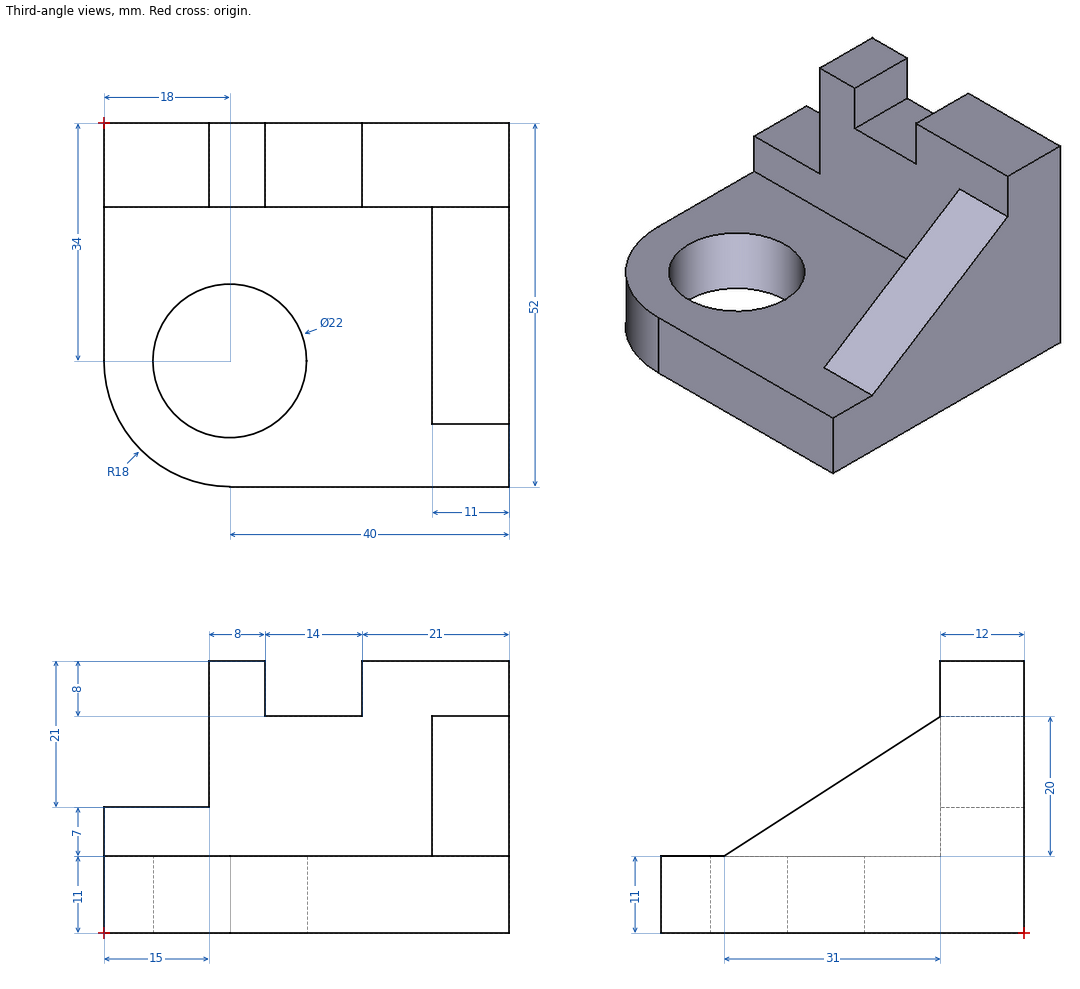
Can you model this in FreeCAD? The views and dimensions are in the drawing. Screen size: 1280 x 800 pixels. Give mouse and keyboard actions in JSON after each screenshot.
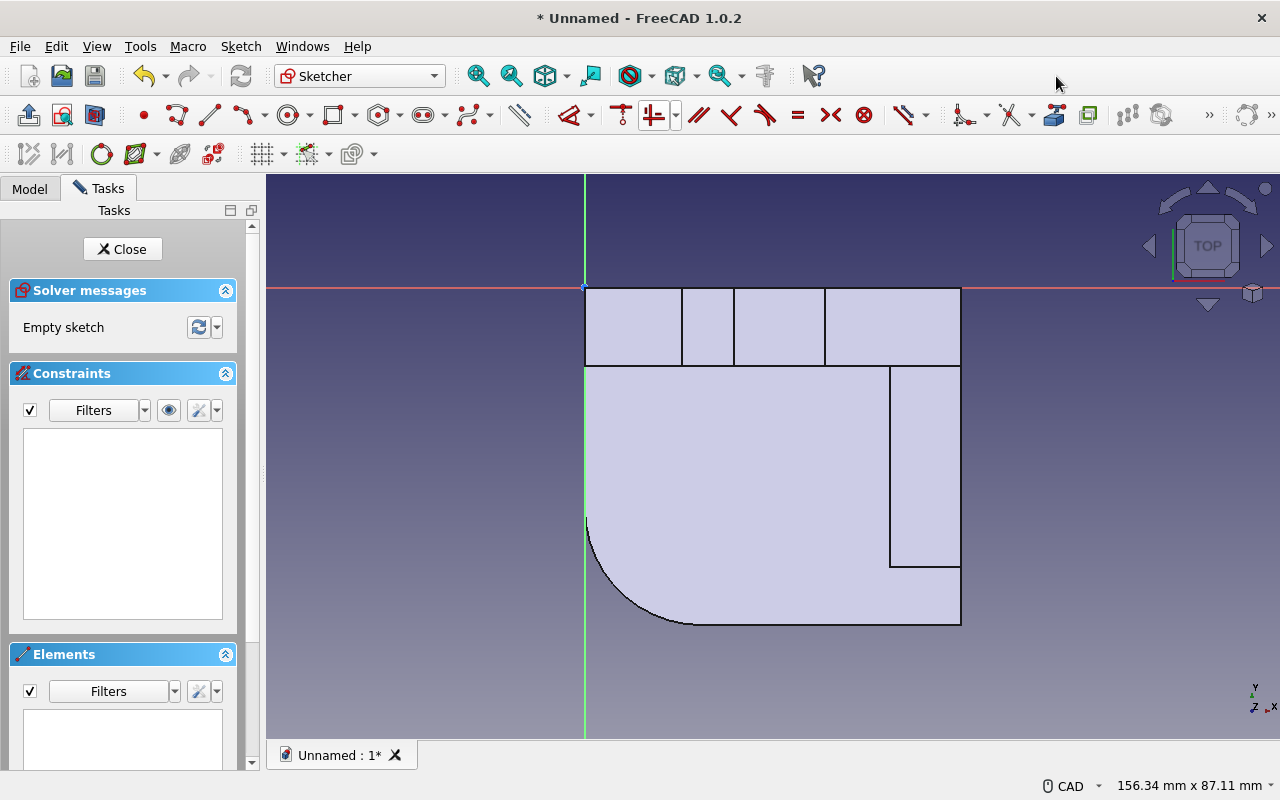
{"action": "left_click", "coordinate": [95, 116]}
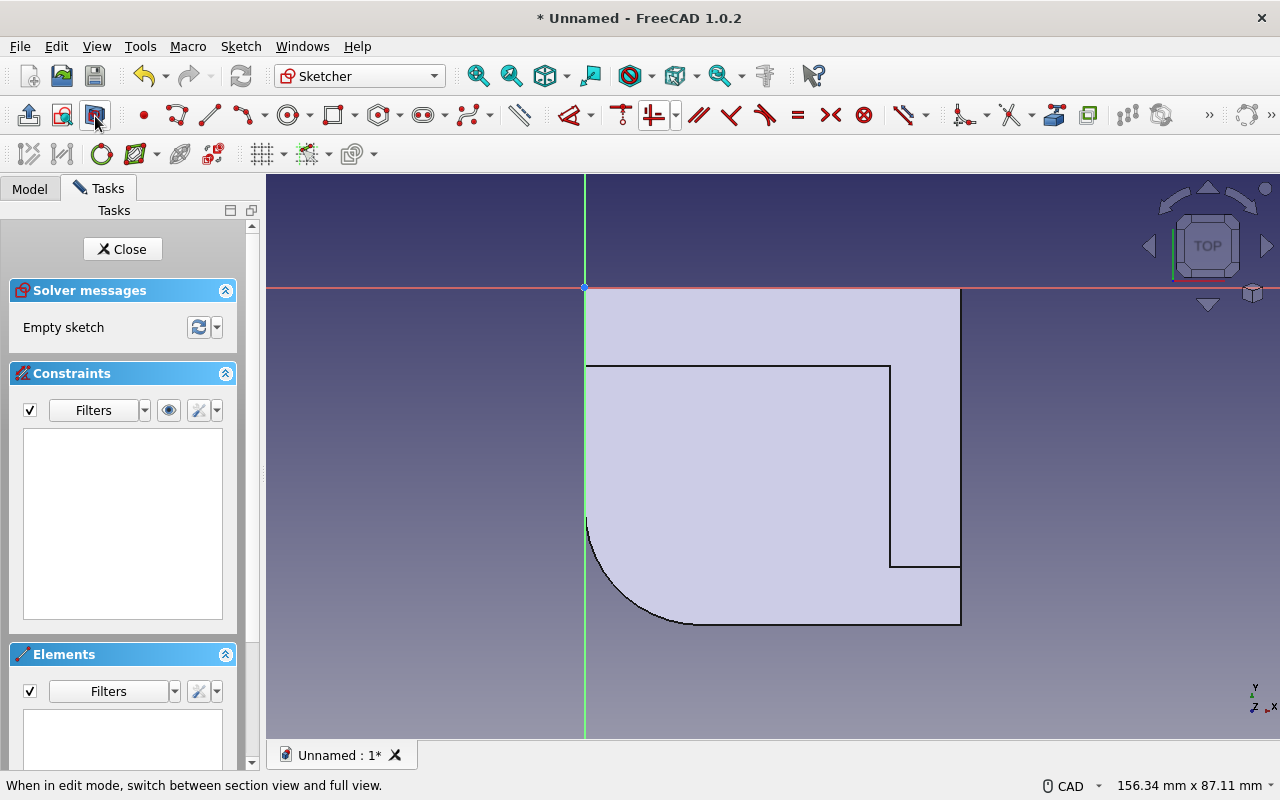
{"action": "left_click", "coordinate": [288, 116]}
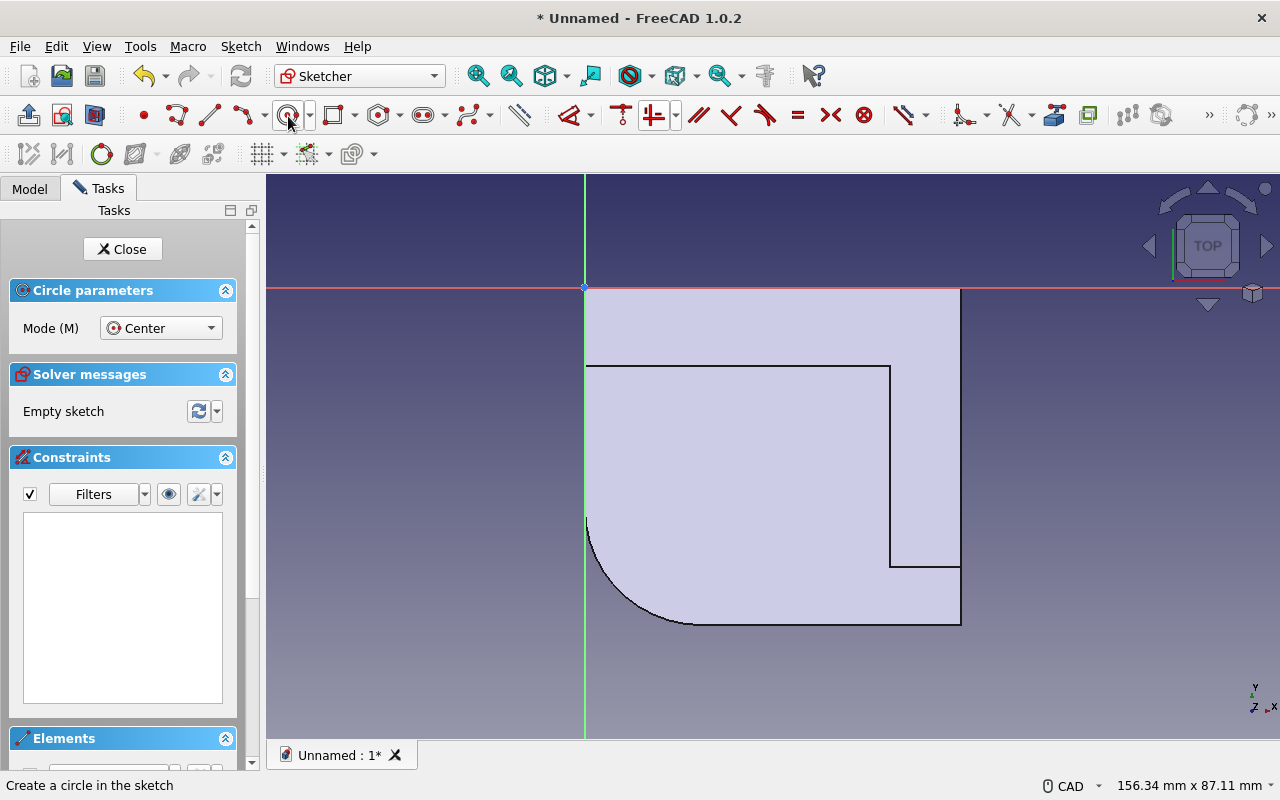
{"action": "left_click", "coordinate": [702, 508]}
{"action": "left_click", "coordinate": [752, 458]}
{"action": "key", "text": "Escape"}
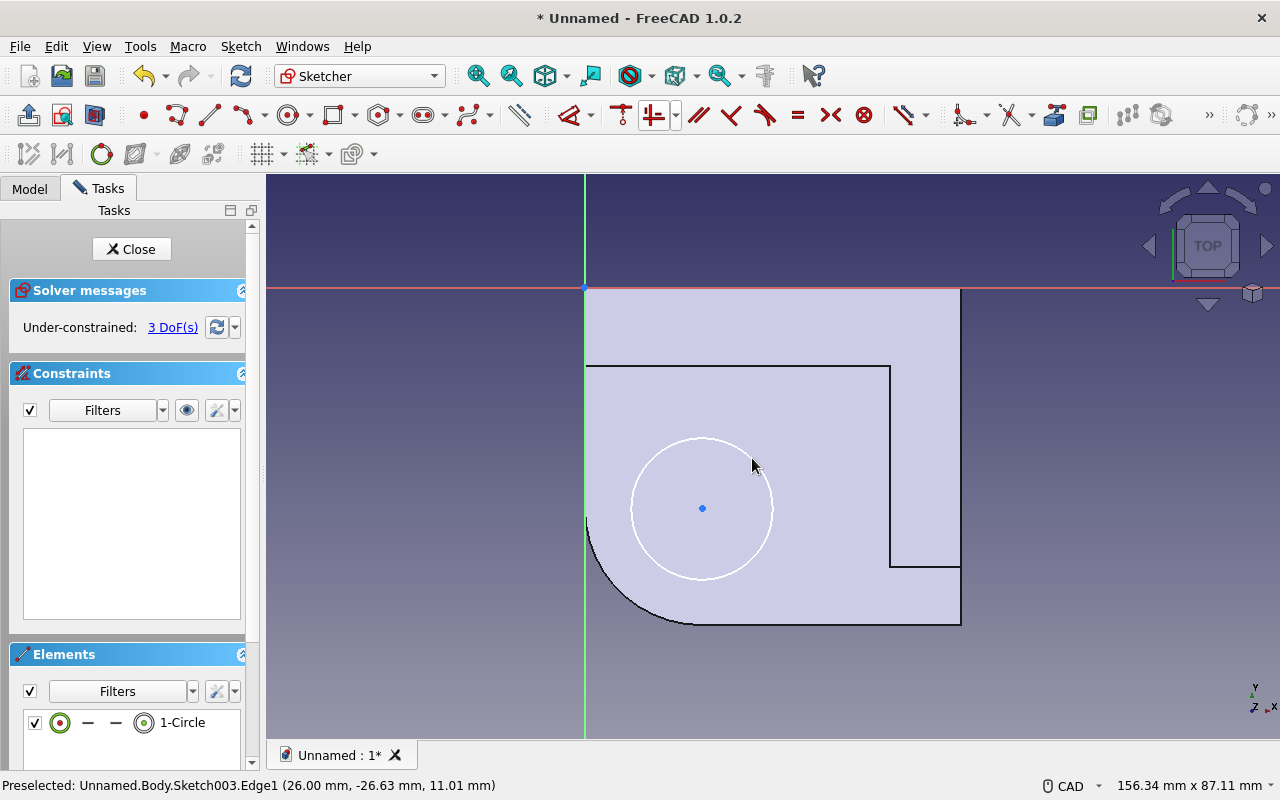
{"action": "left_click", "coordinate": [568, 116]}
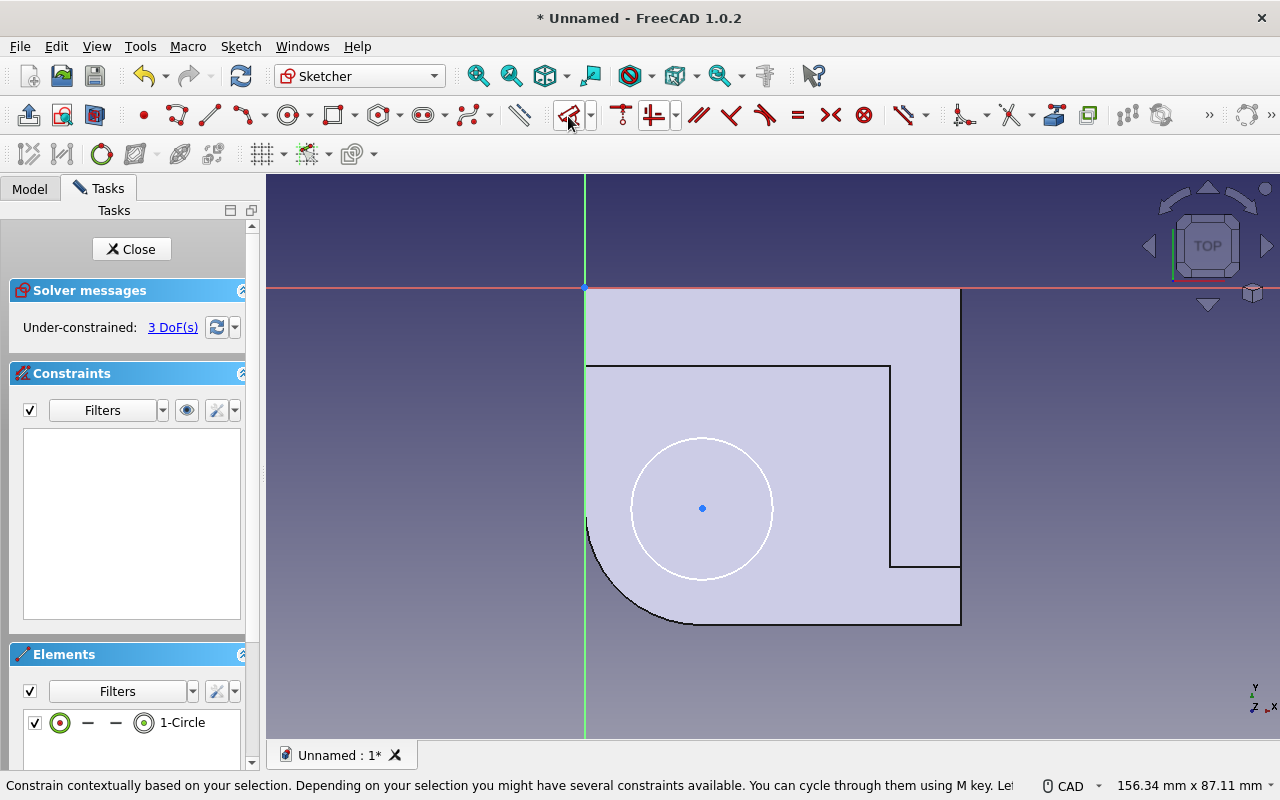
{"action": "left_click", "coordinate": [752, 459]}
{"action": "left_click", "coordinate": [775, 436]}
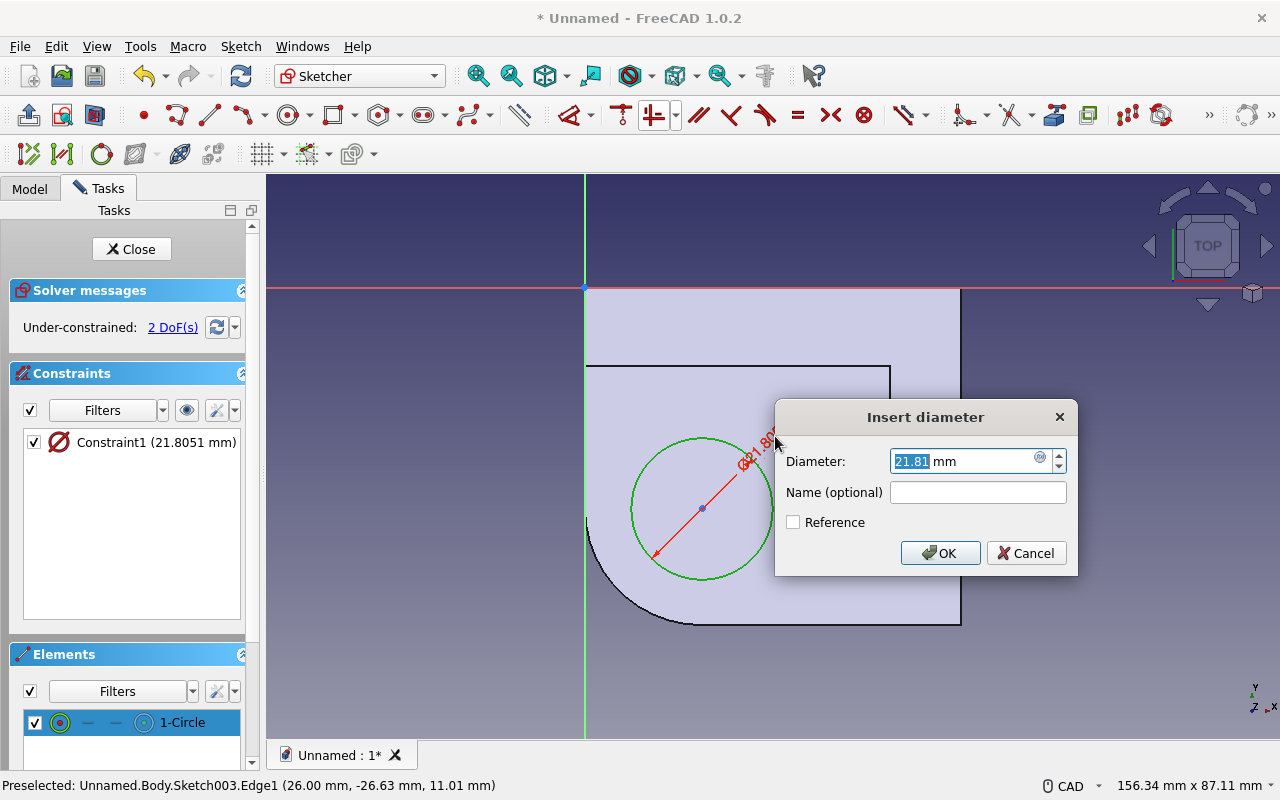
{"action": "type", "text": "22"}
{"action": "key", "text": "Return"}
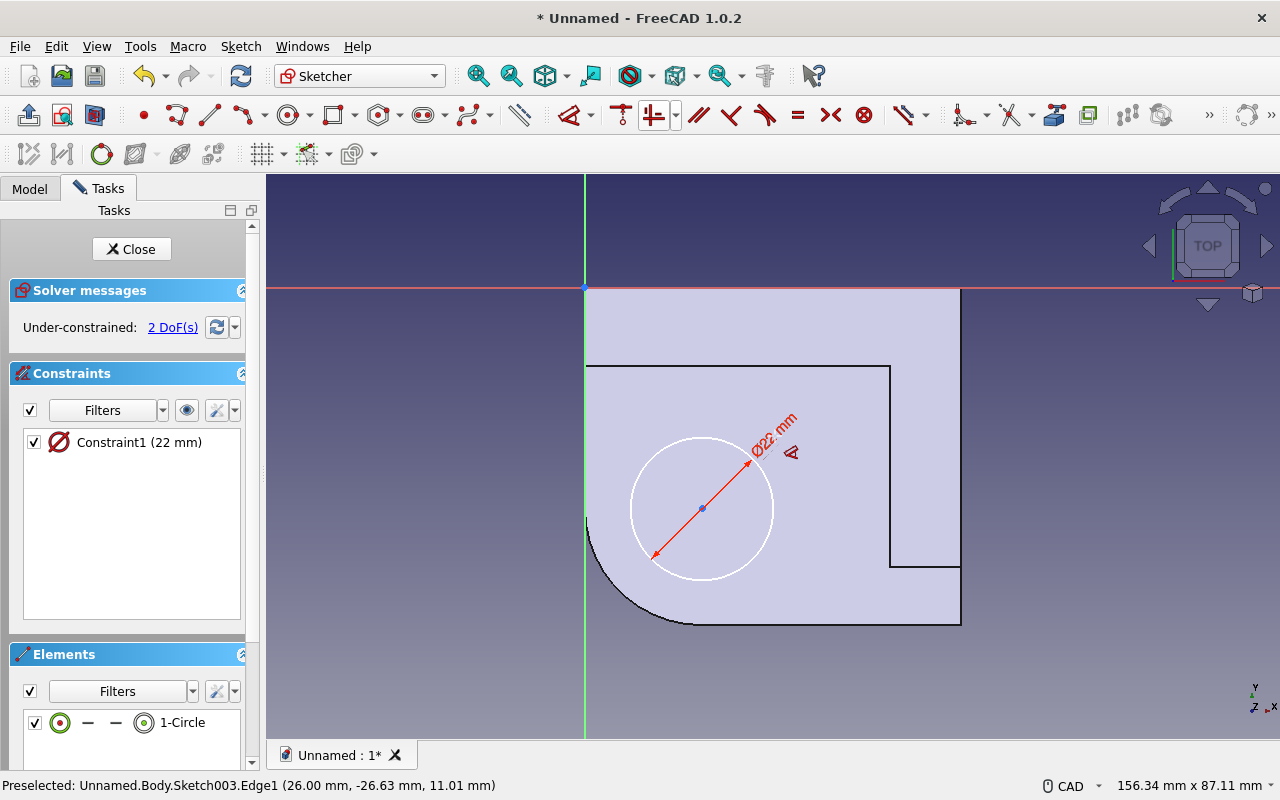
{"action": "left_click", "coordinate": [702, 509]}
{"action": "left_click", "coordinate": [643, 254]}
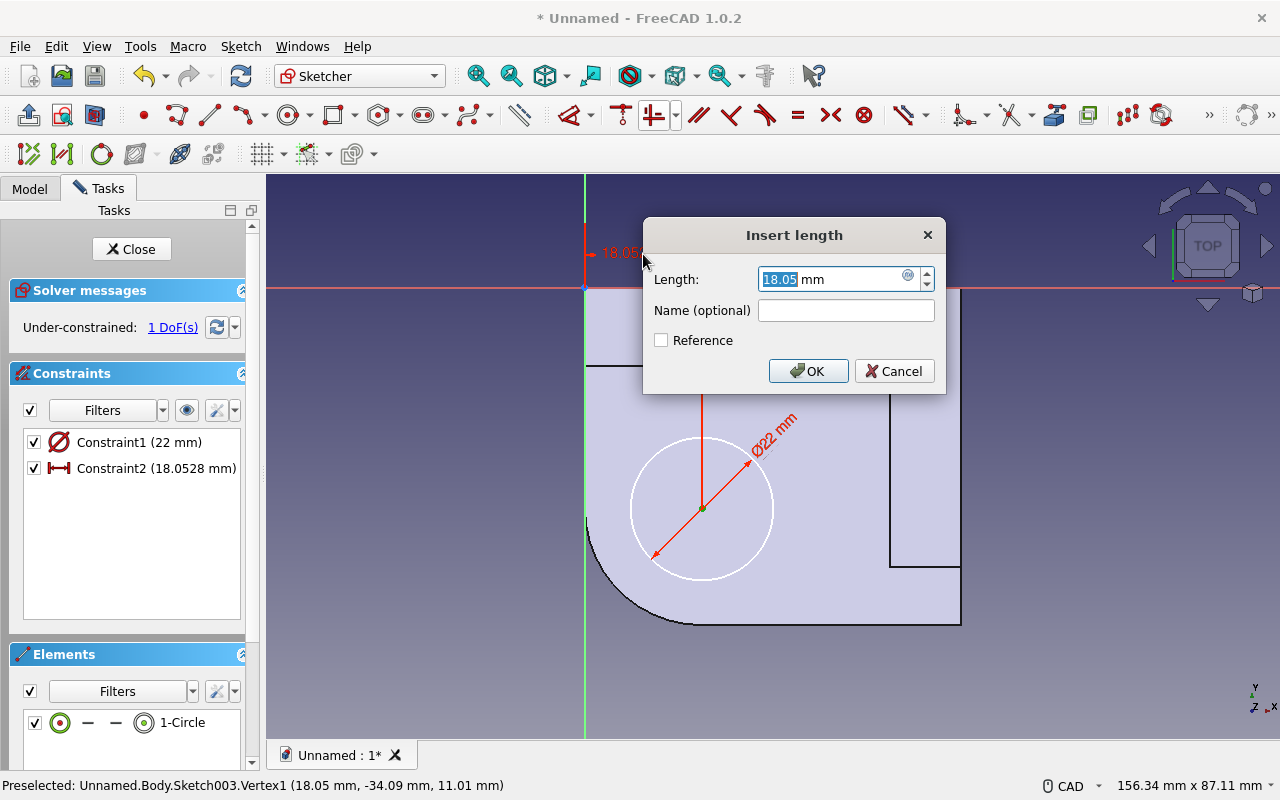
{"action": "type", "text": "18"}
{"action": "key", "text": "Return"}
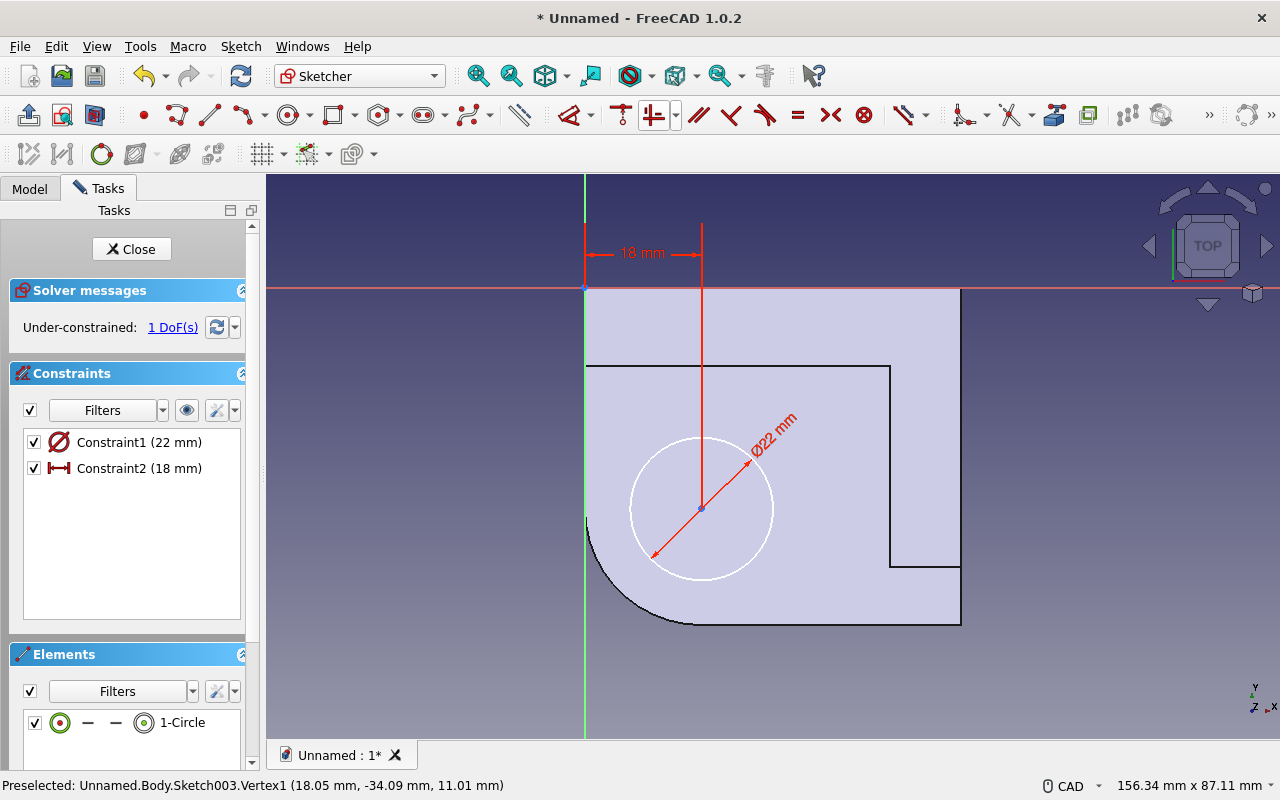
{"action": "left_click", "coordinate": [702, 509]}
{"action": "left_click", "coordinate": [551, 398]}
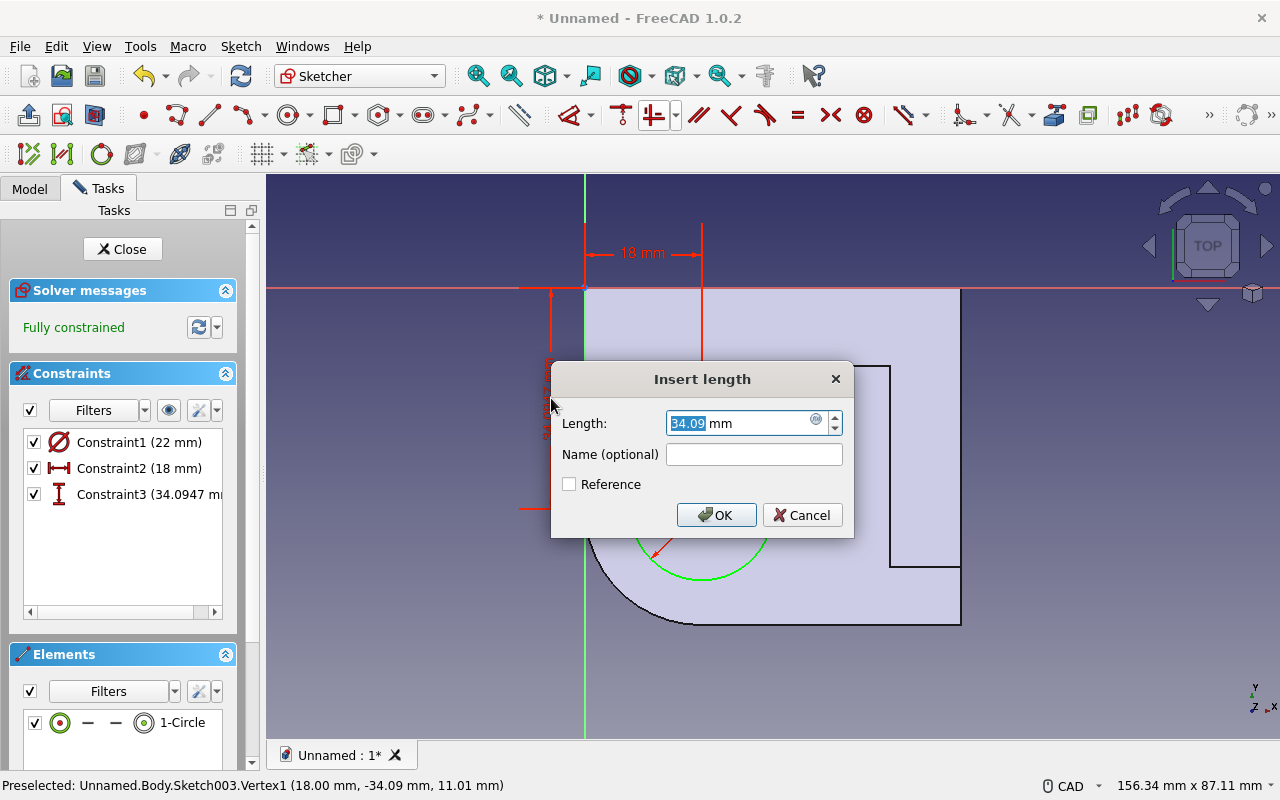
{"action": "type", "text": "34"}
{"action": "key", "text": "Return"}
{"action": "key", "text": "Escape"}